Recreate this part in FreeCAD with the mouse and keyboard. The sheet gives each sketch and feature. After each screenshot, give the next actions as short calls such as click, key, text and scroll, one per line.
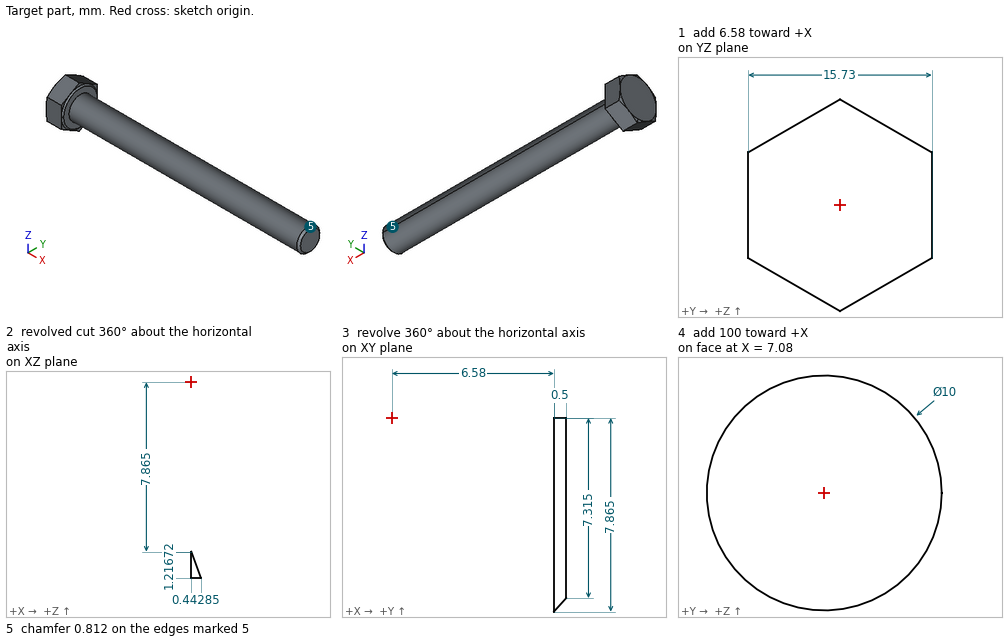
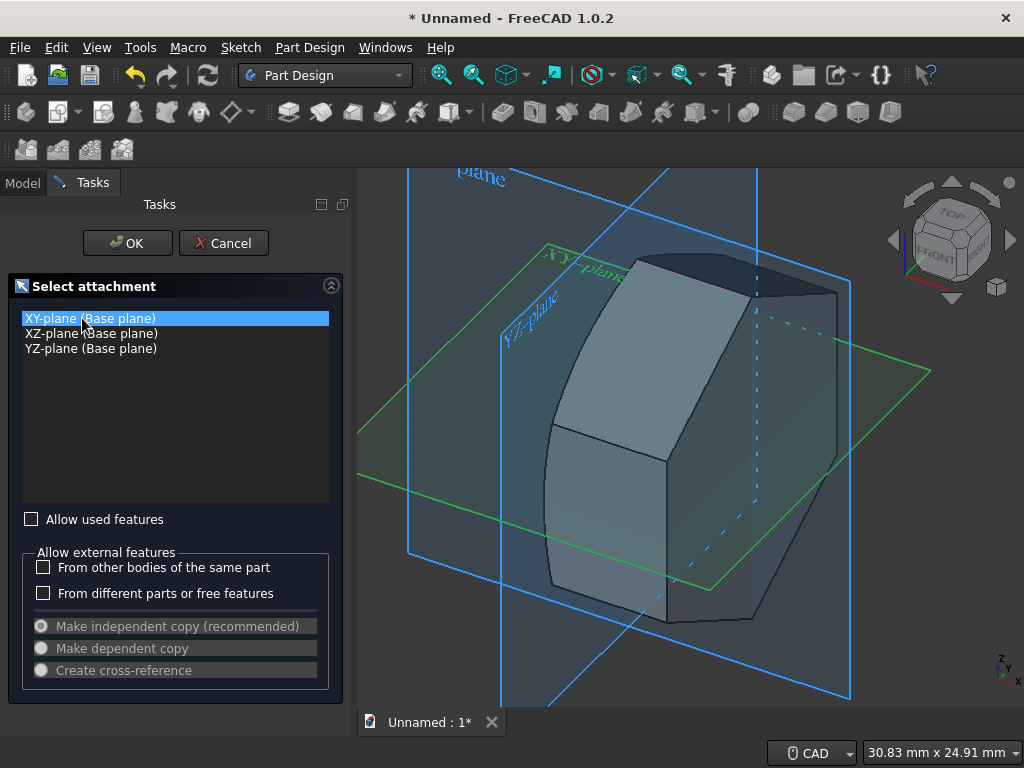
click(128, 243)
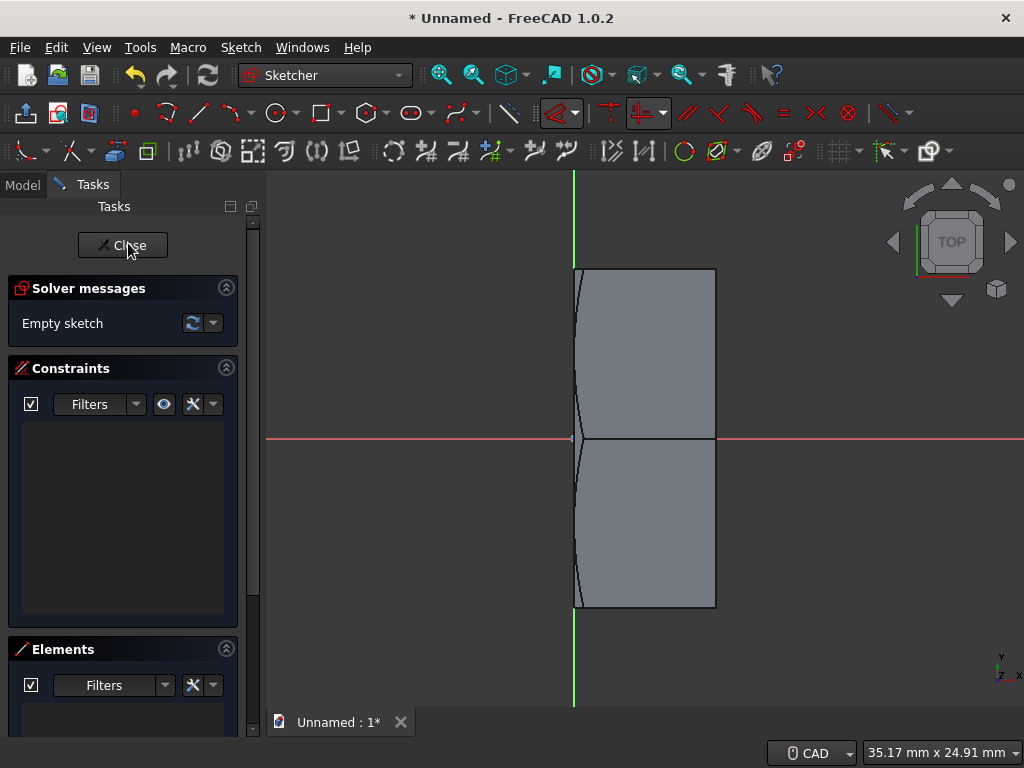
click(90, 114)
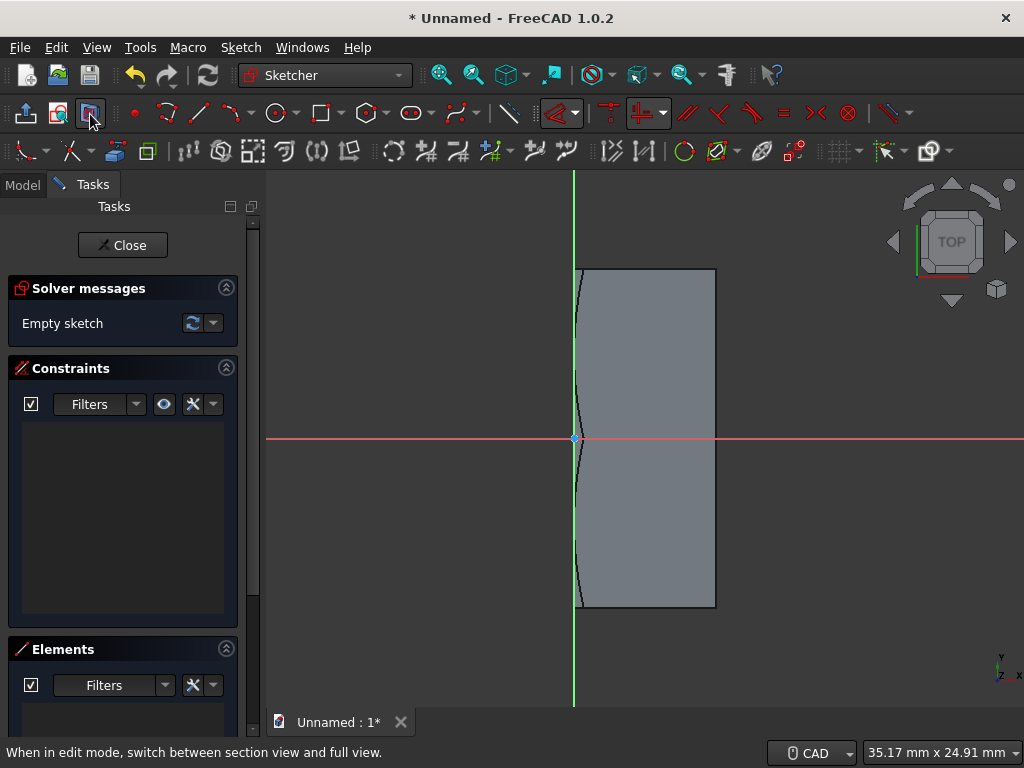
scroll(740, 626, up, 3)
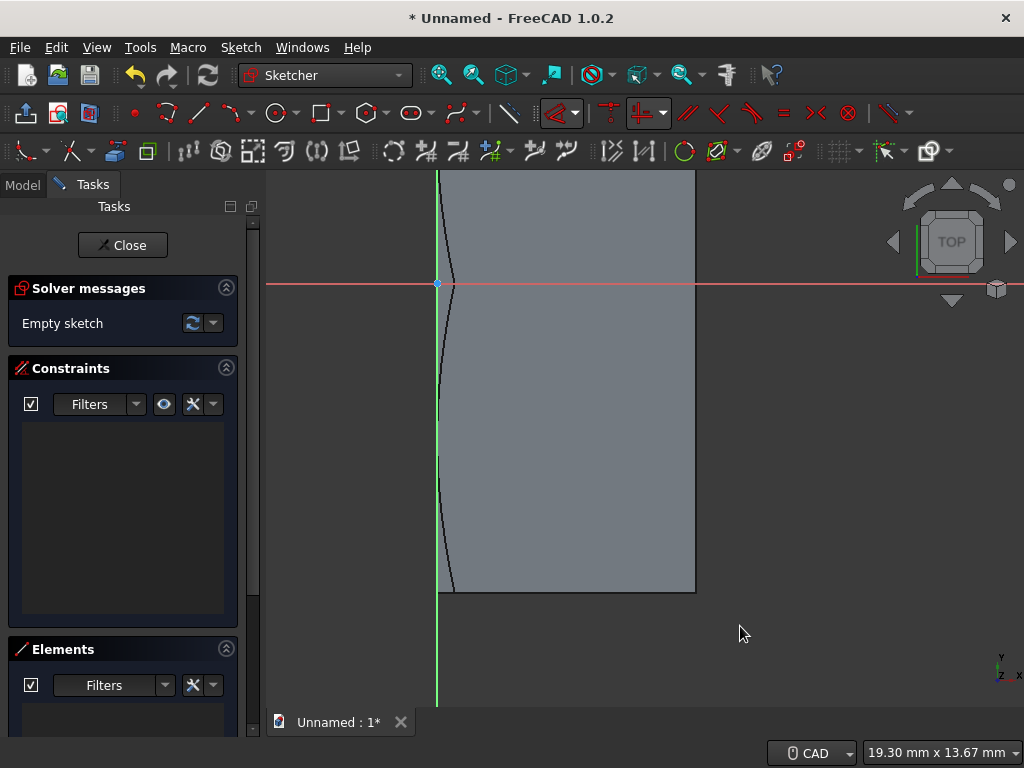
click(168, 114)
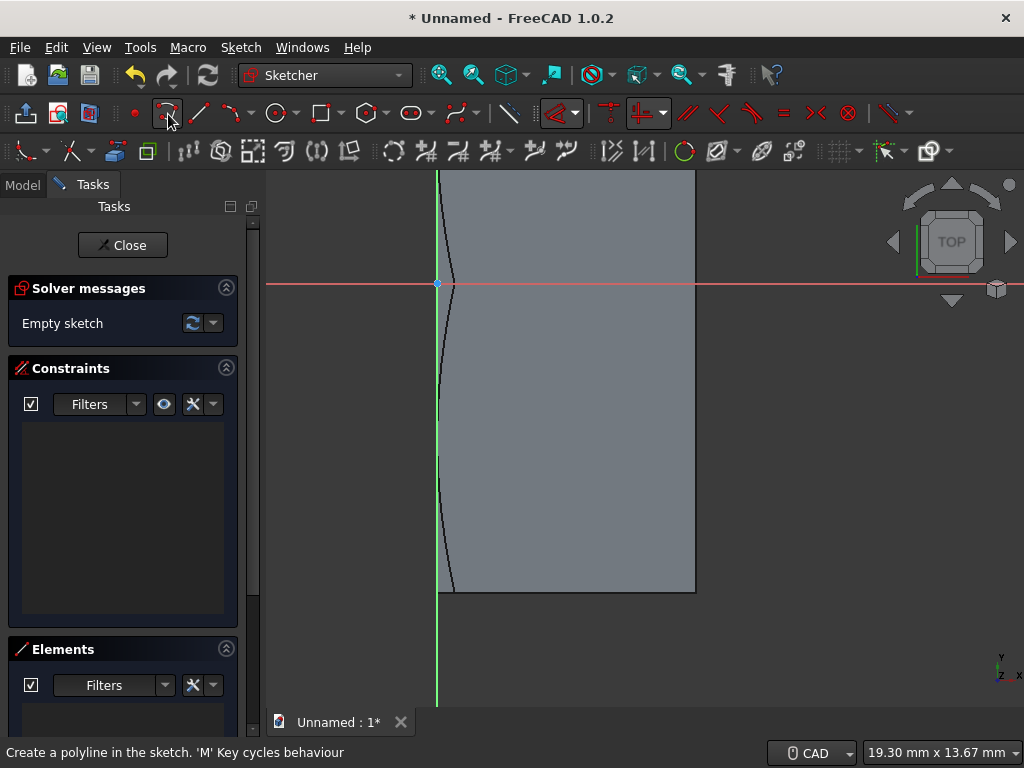
click(696, 284)
click(696, 593)
click(715, 571)
click(715, 293)
click(696, 284)
key(Escape)
key(Escape)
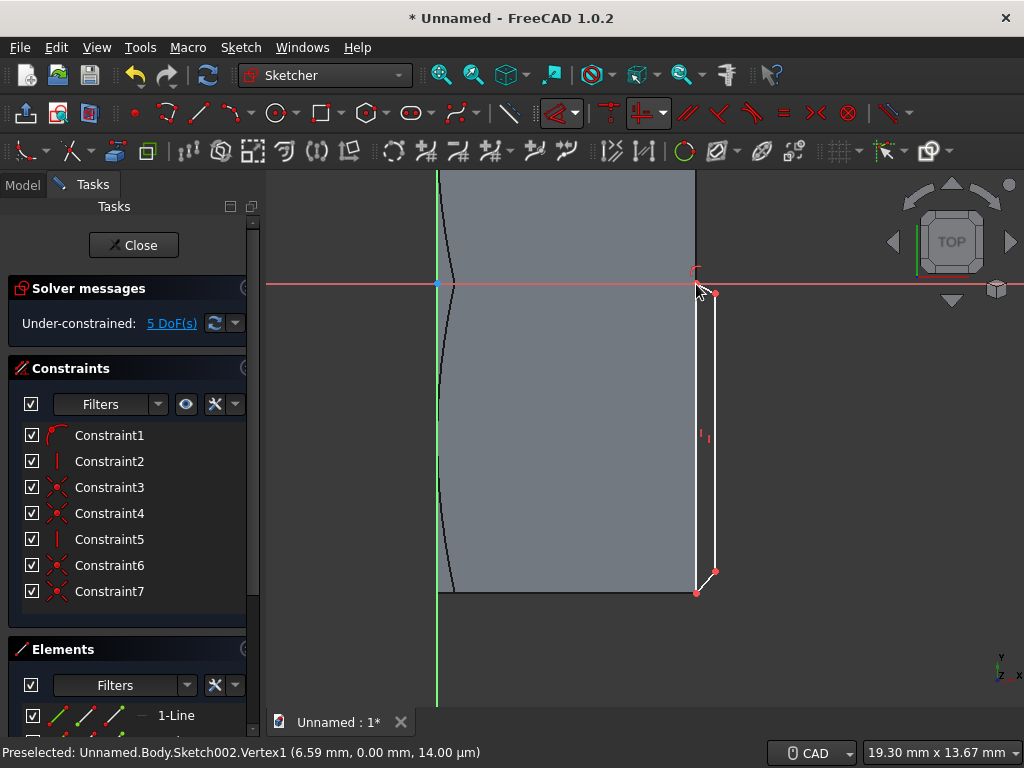
scroll(709, 291, up, 4)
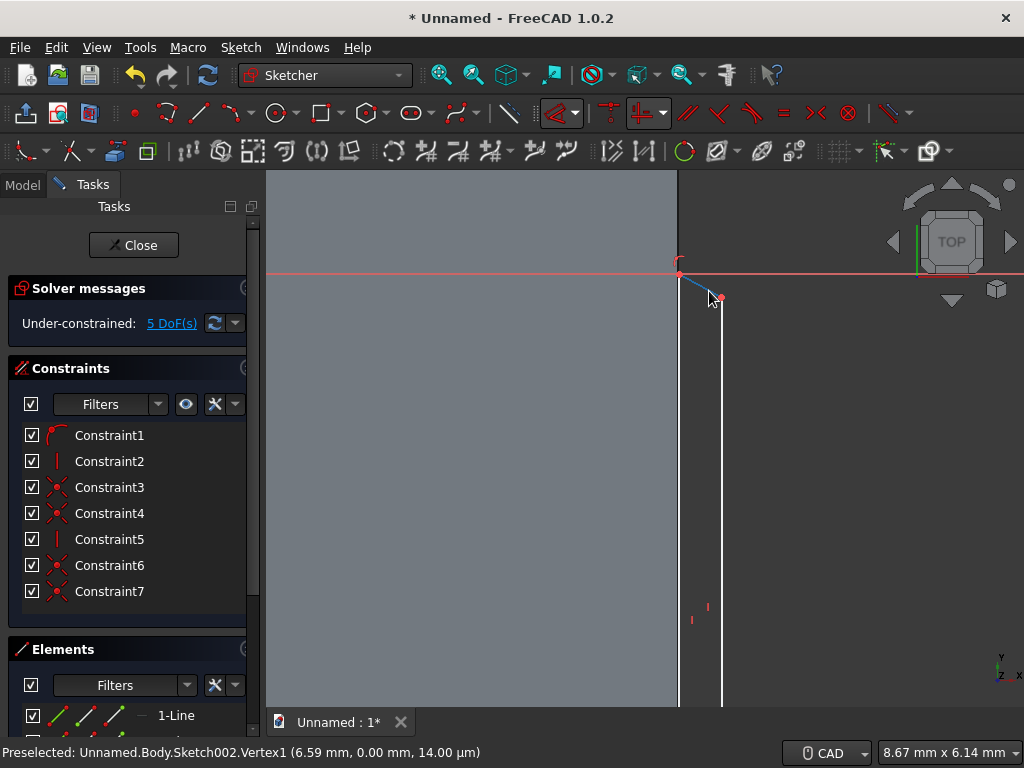
click(709, 290)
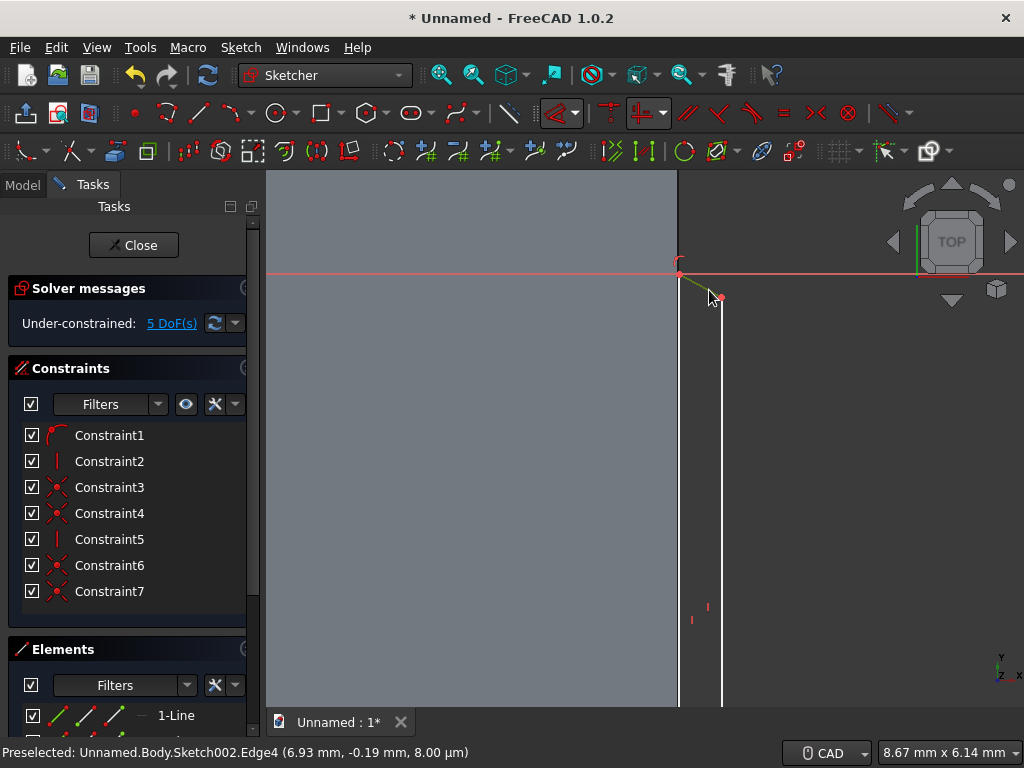
key(h)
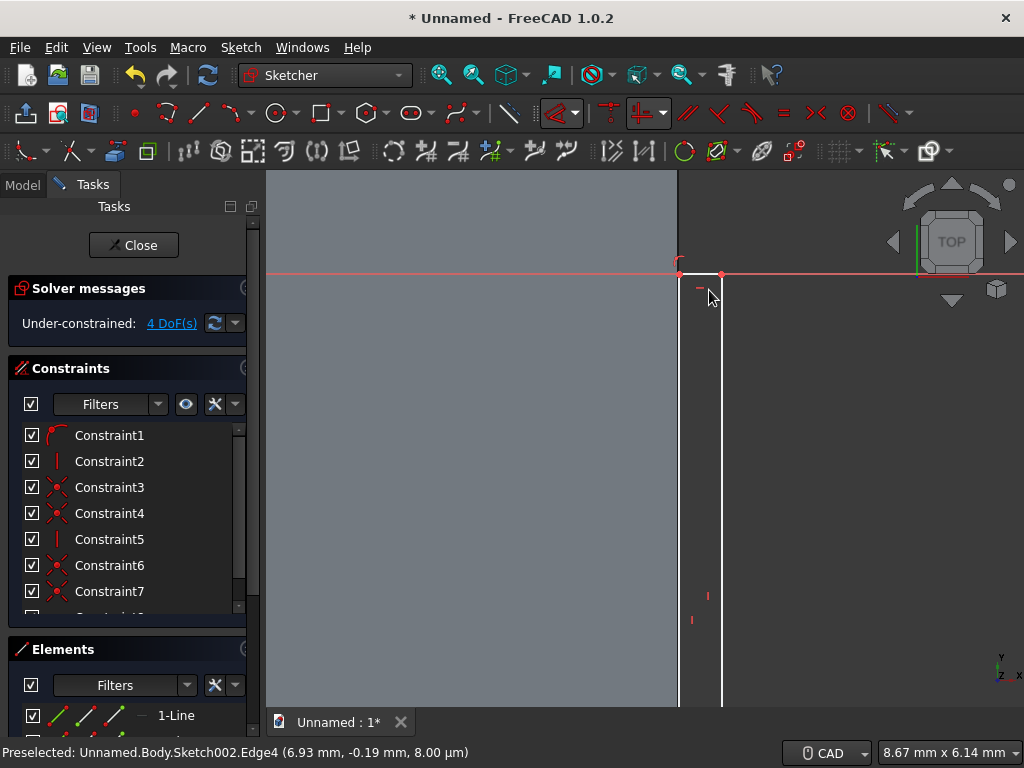
key(d)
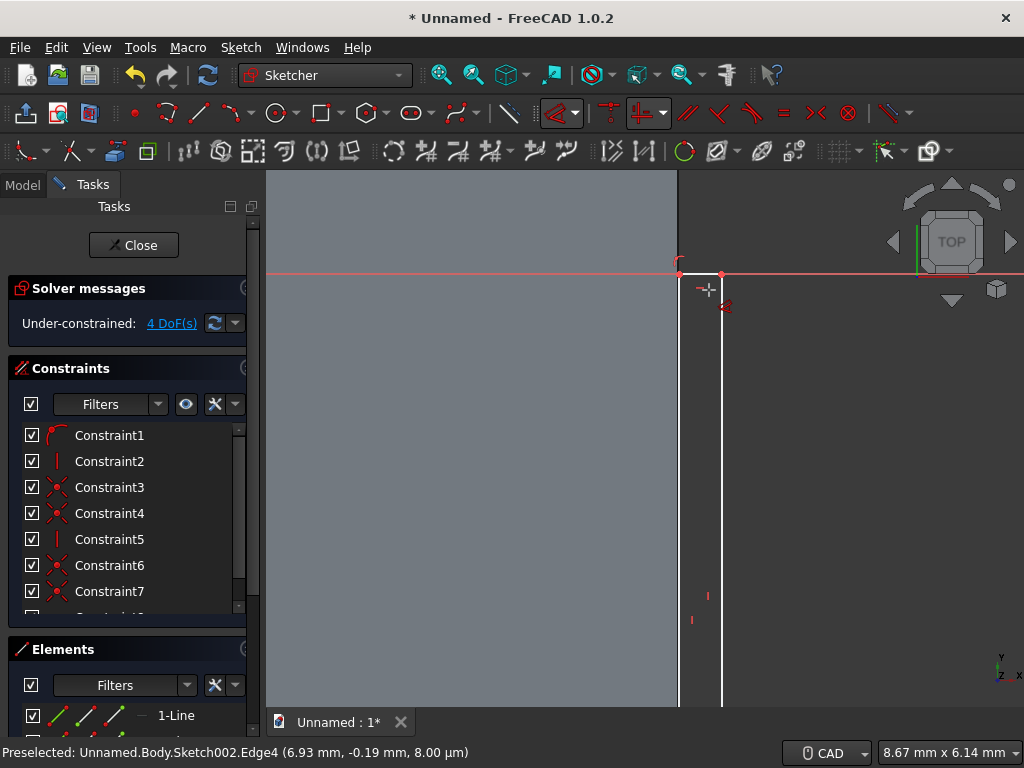
click(709, 274)
click(700, 240)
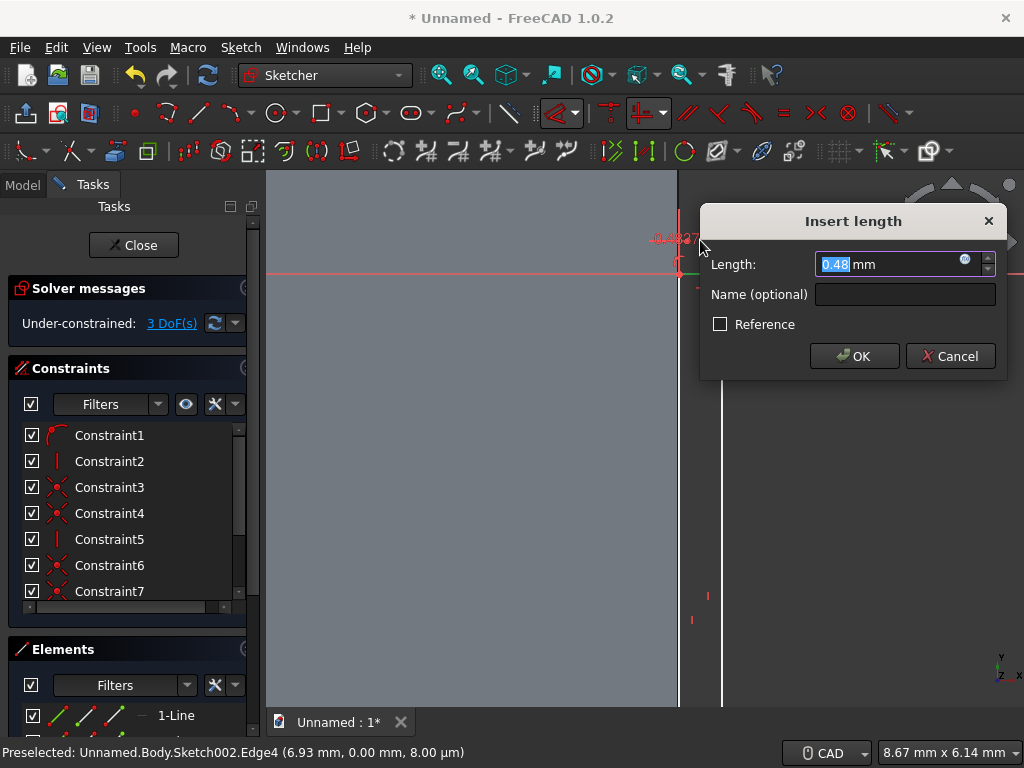
text(0.5)
key(Return)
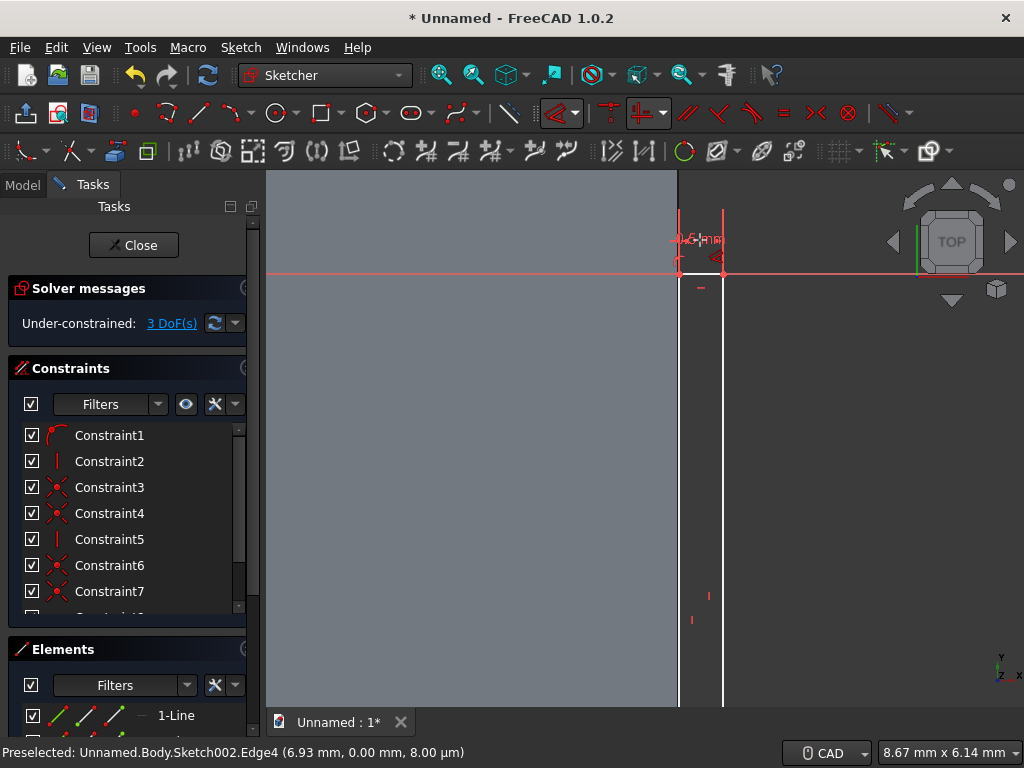
click(679, 482)
click(645, 477)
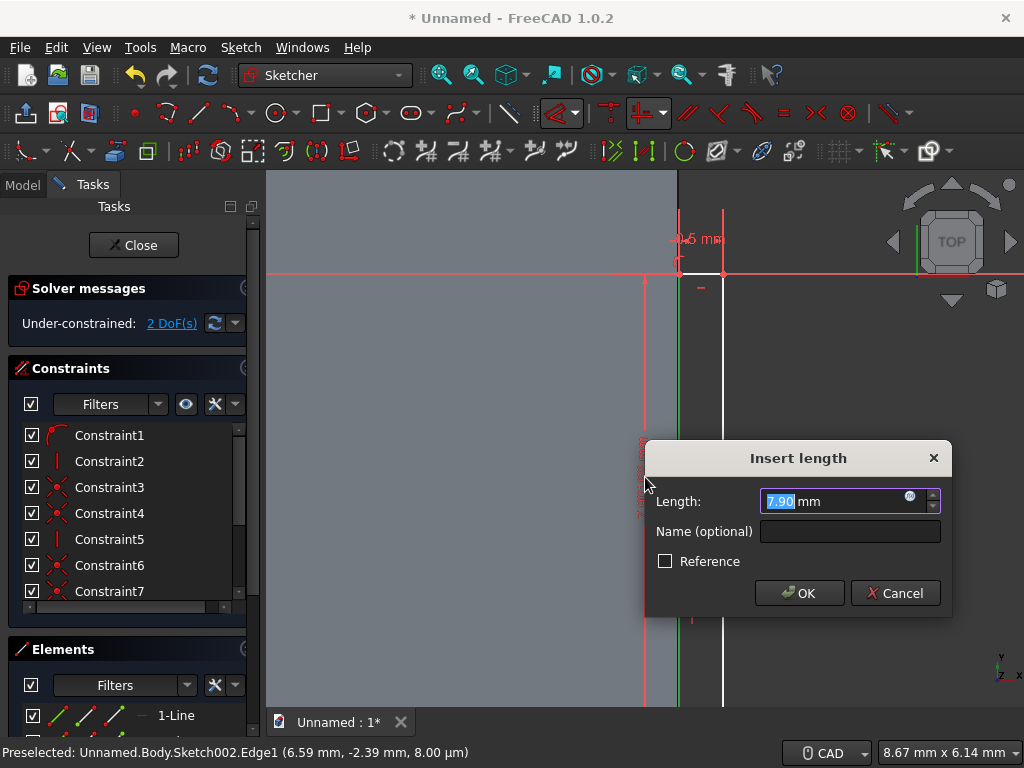
text(7.865)
key(Return)